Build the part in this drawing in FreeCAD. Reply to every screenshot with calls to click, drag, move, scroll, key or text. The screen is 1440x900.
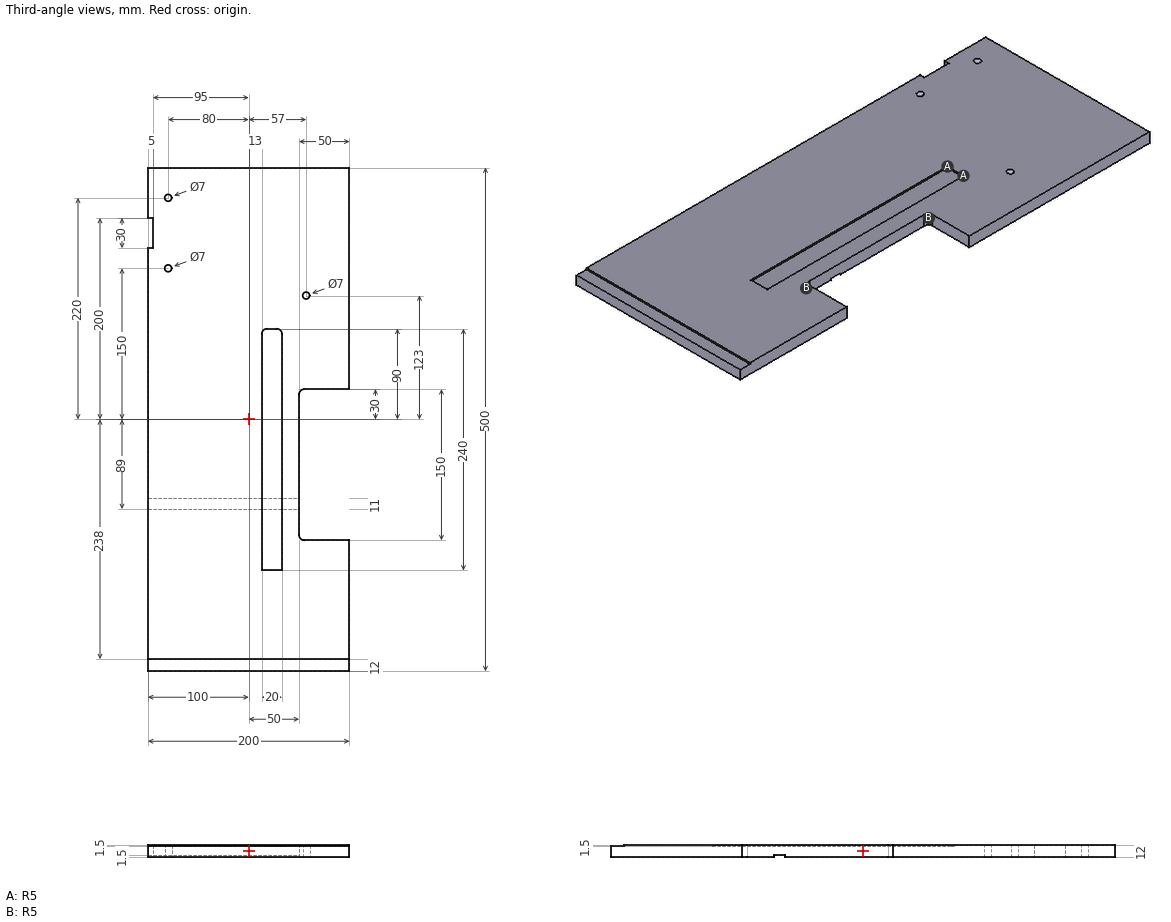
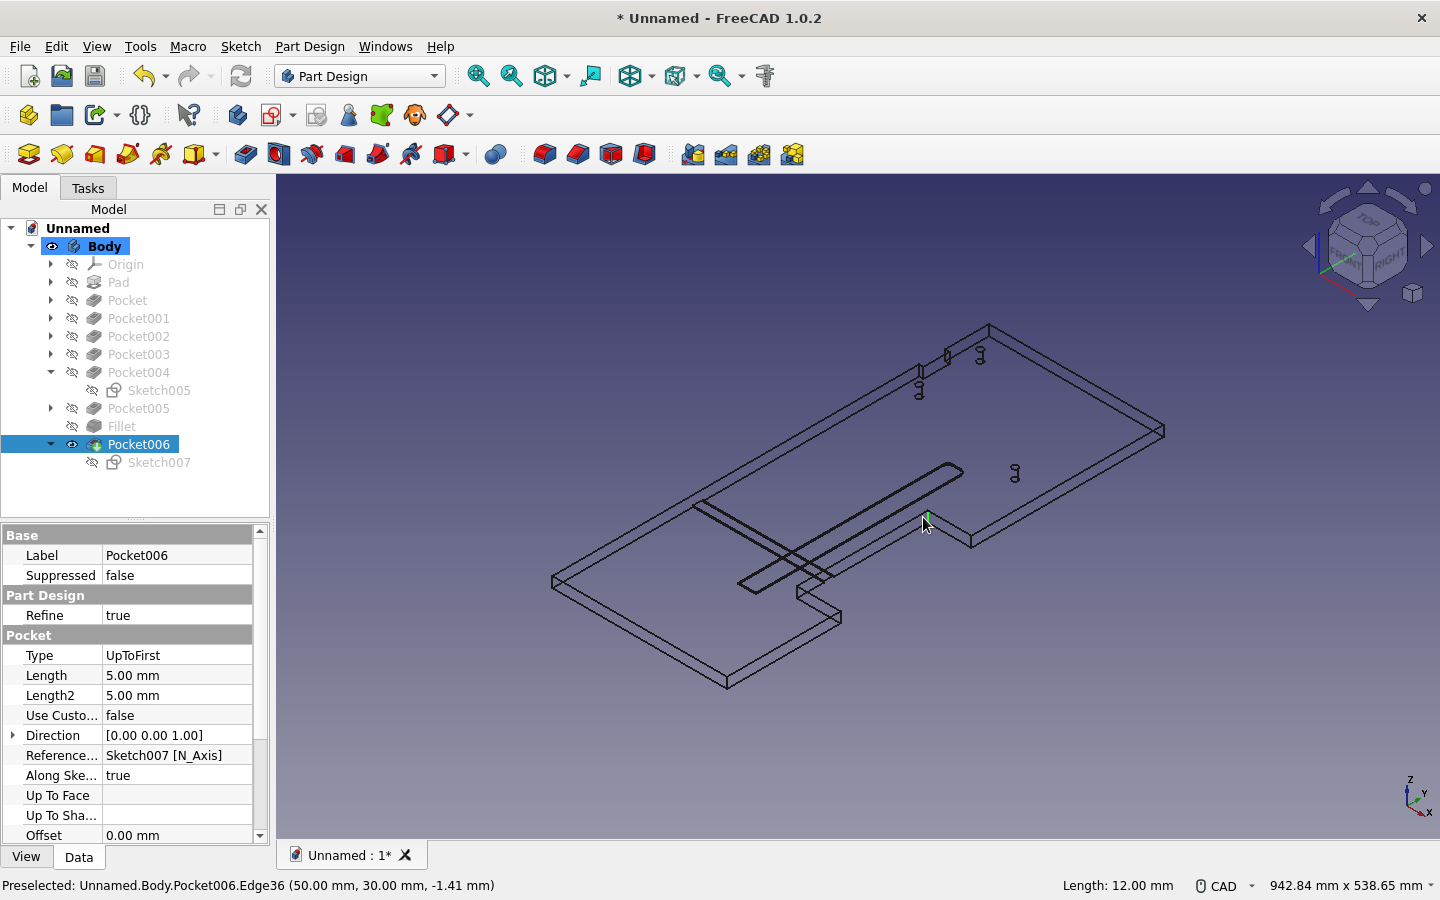
click(797, 594, ctrl)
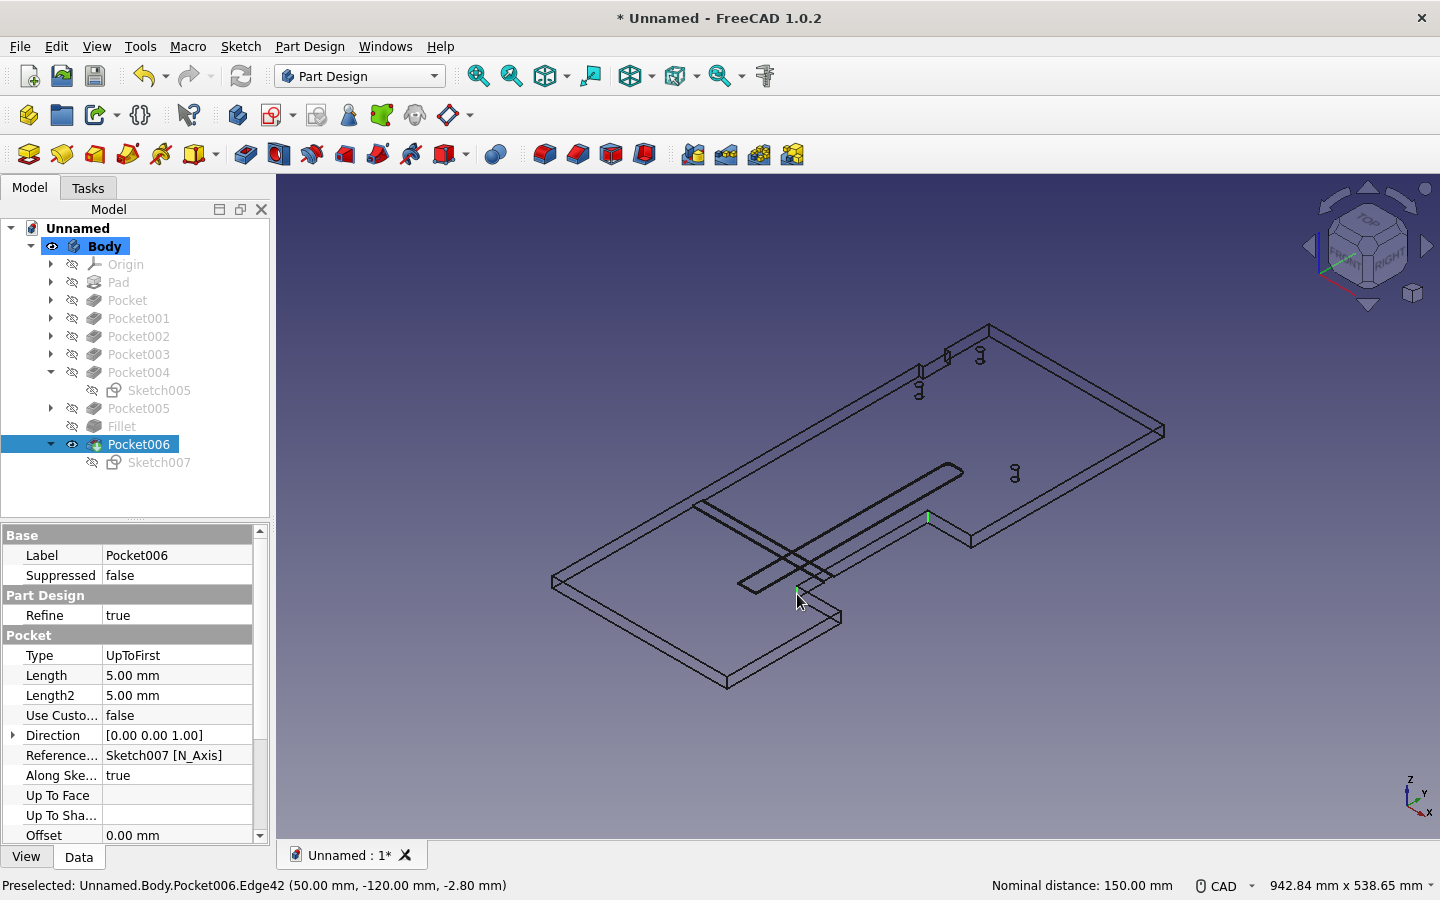
key(v)
key(1)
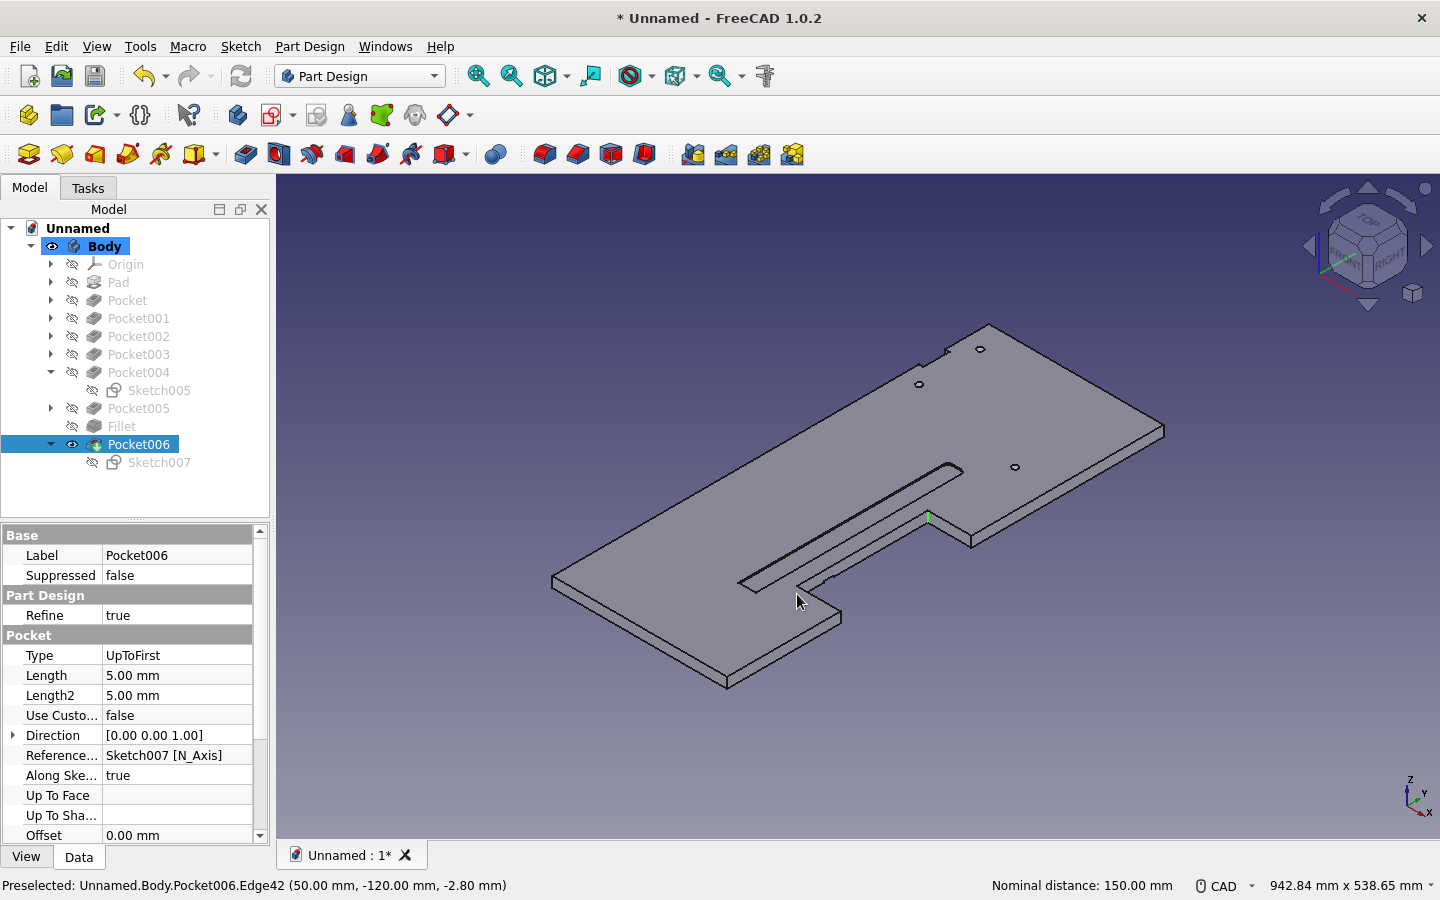
click(545, 154)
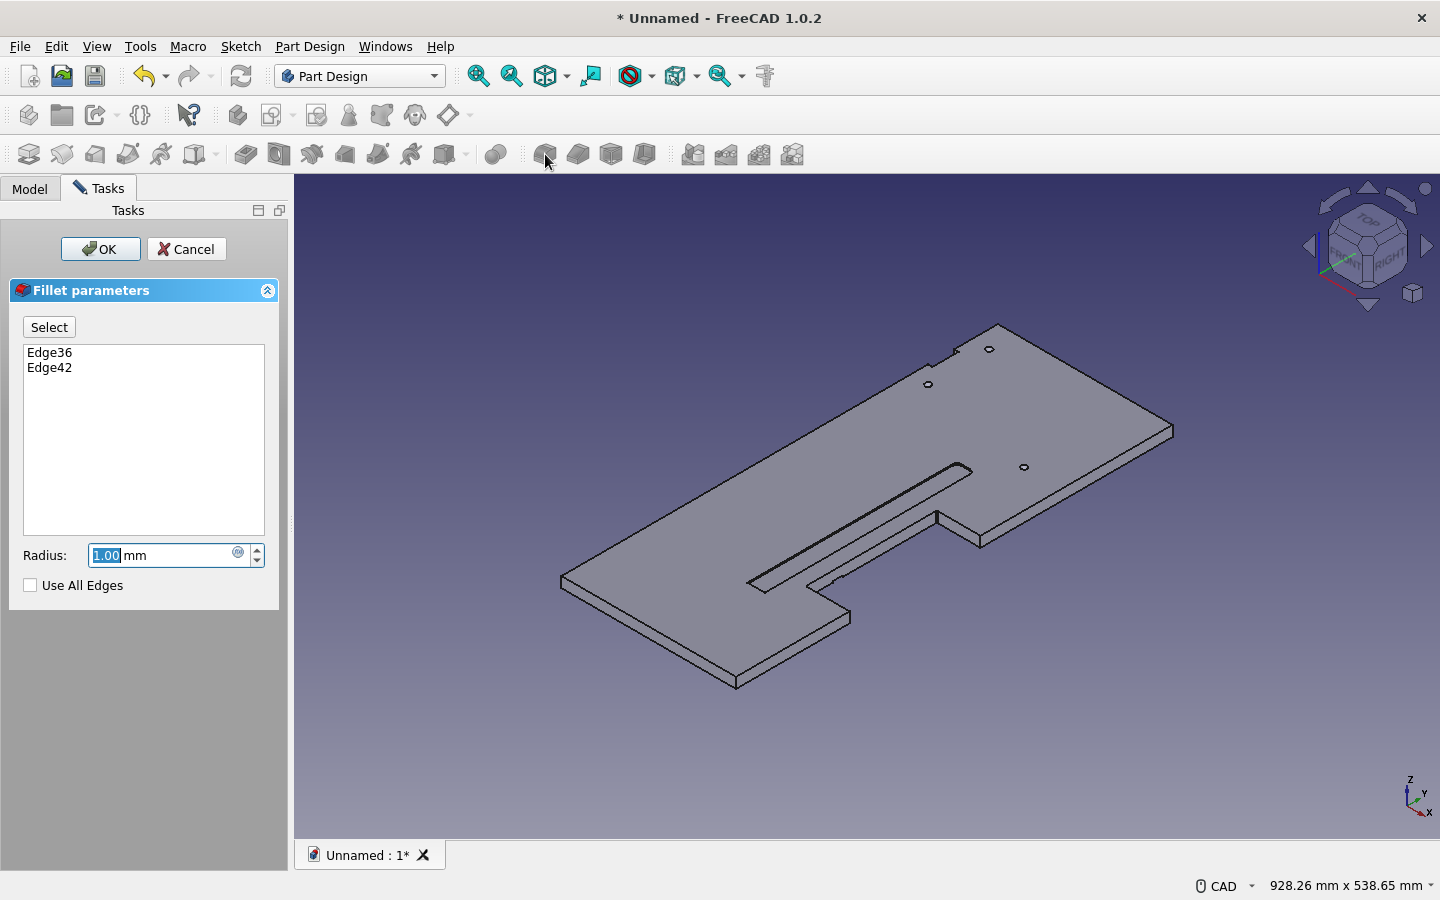
text(5)
key(Tab)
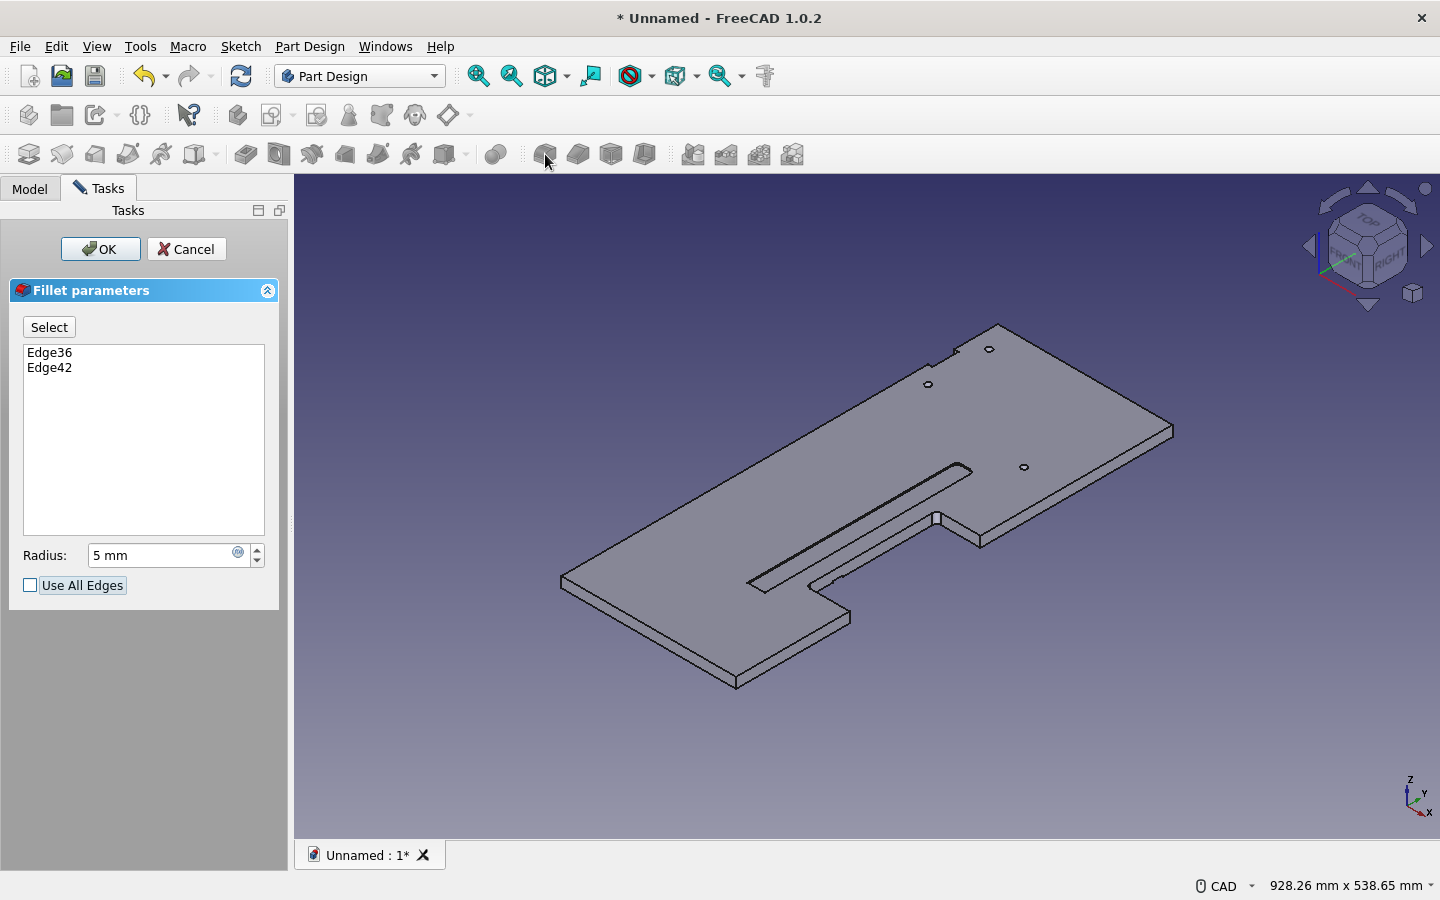
click(101, 249)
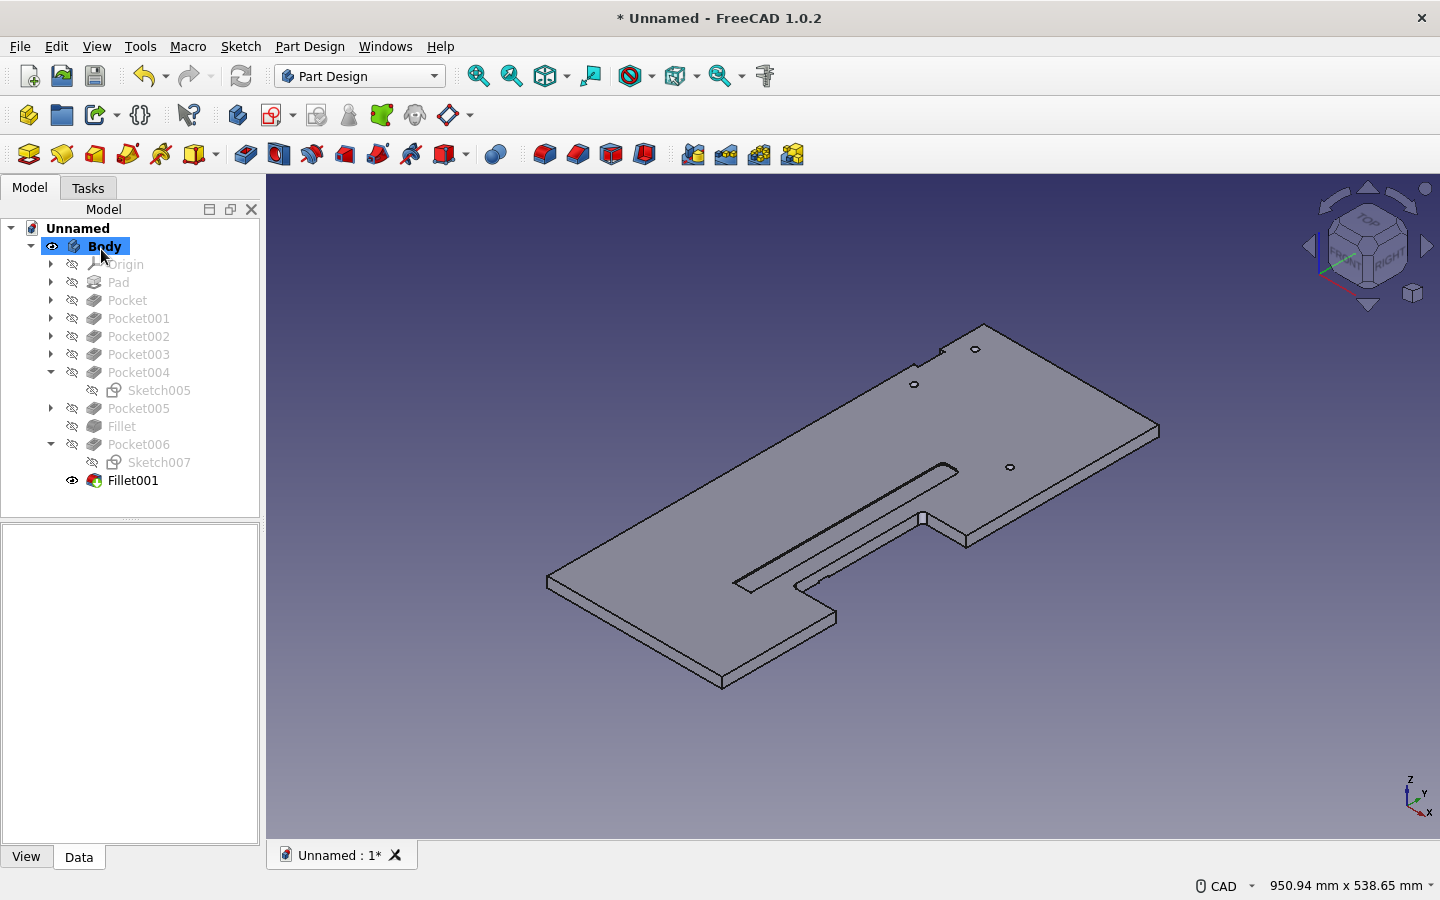
click(978, 427)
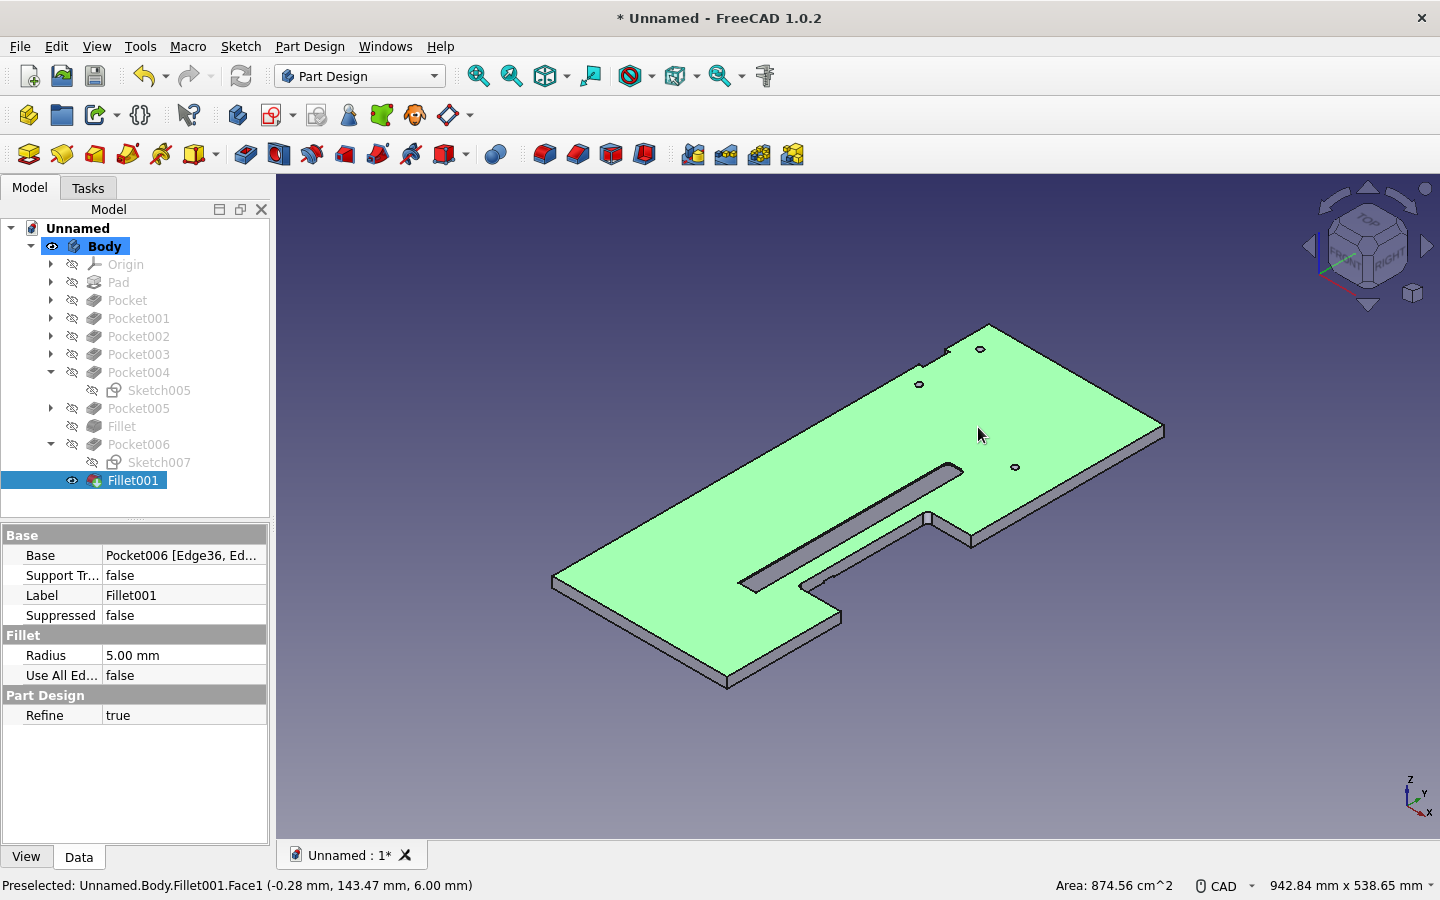
click(270, 116)